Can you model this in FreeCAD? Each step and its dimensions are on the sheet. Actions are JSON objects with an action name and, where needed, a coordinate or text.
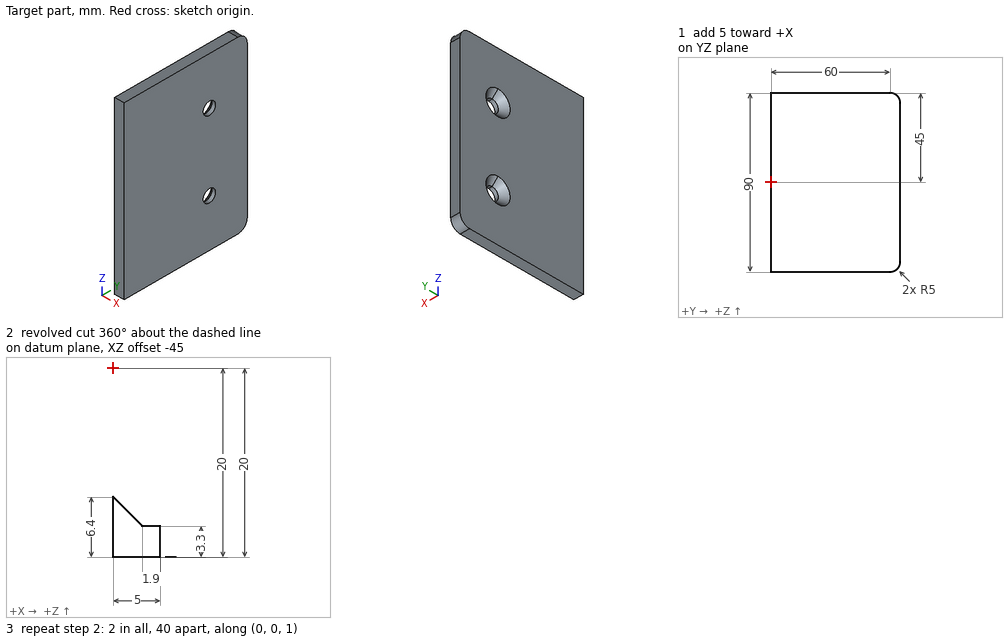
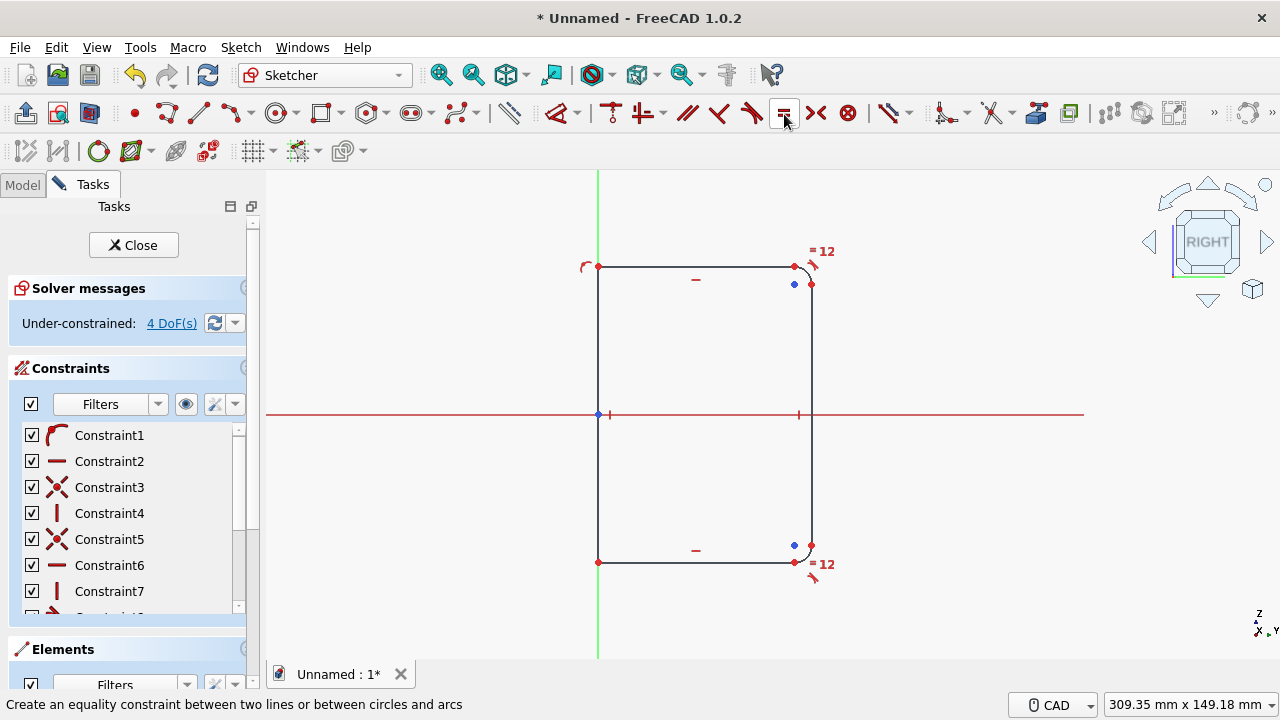
{"action": "left_click", "coordinate": [556, 114]}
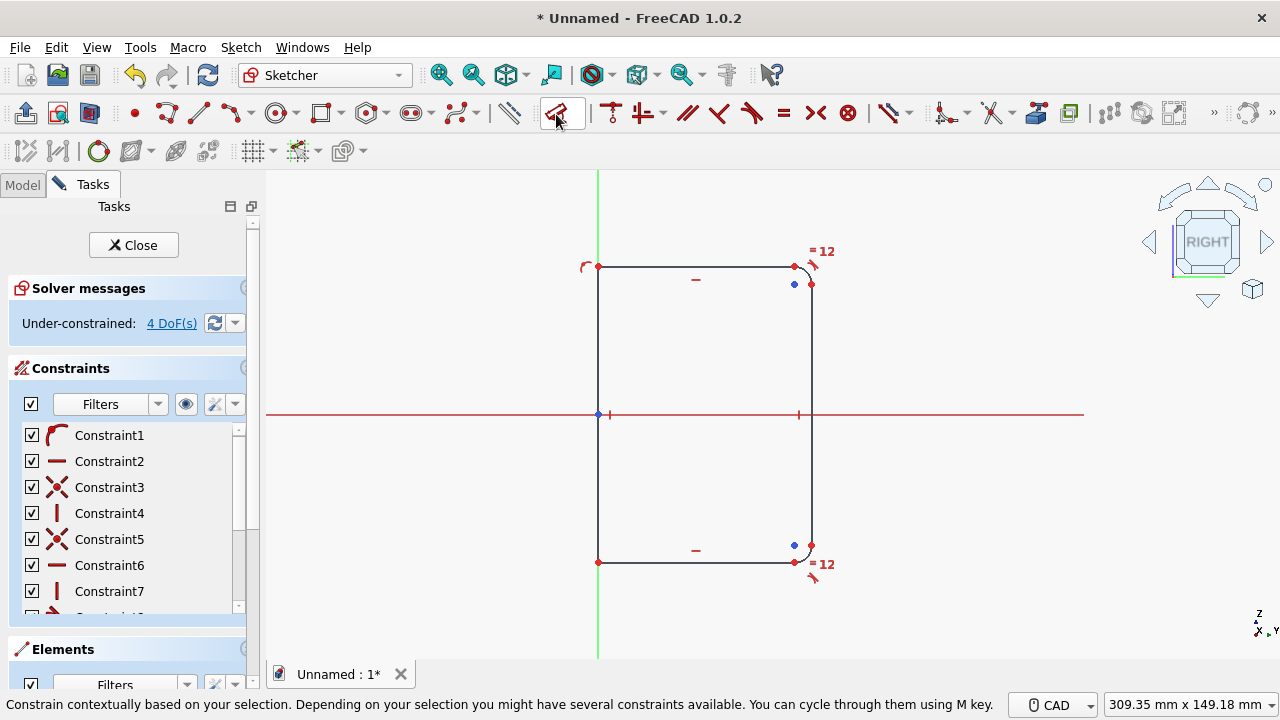
{"action": "scroll", "coordinate": [807, 558], "scroll_direction": "up", "scroll_amount": 5}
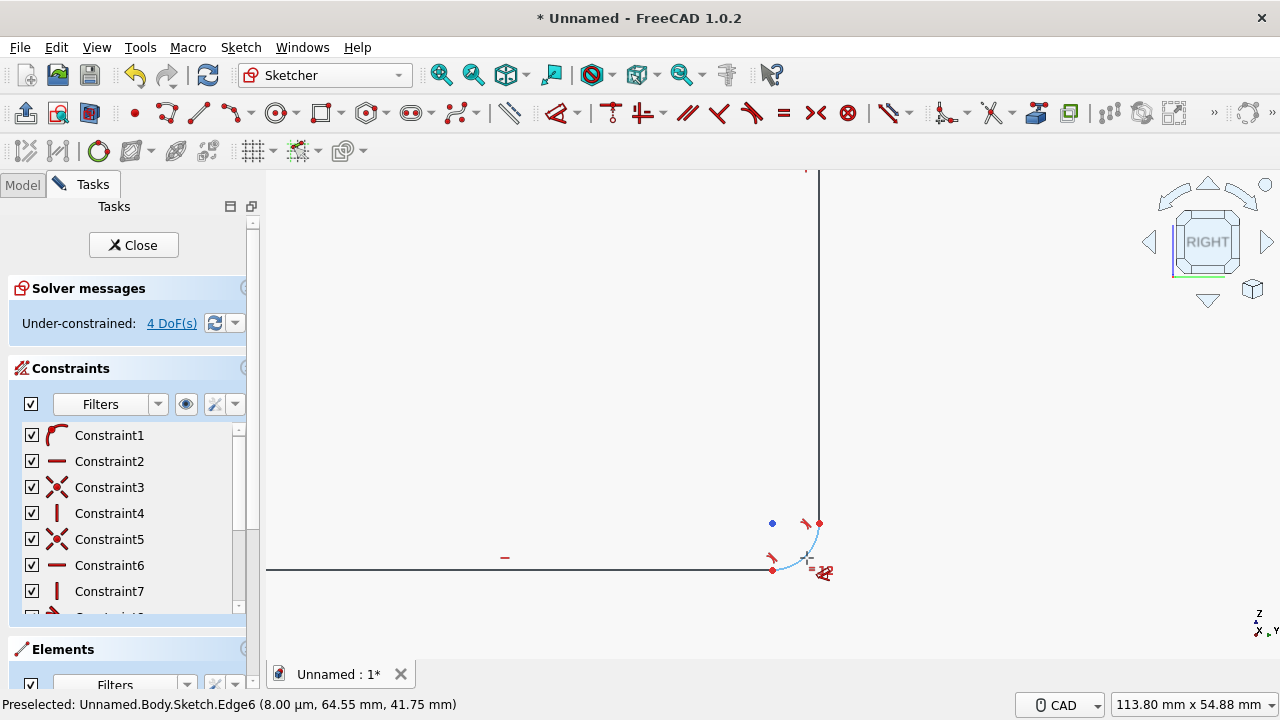
{"action": "left_click", "coordinate": [805, 556]}
{"action": "left_click", "coordinate": [828, 579]}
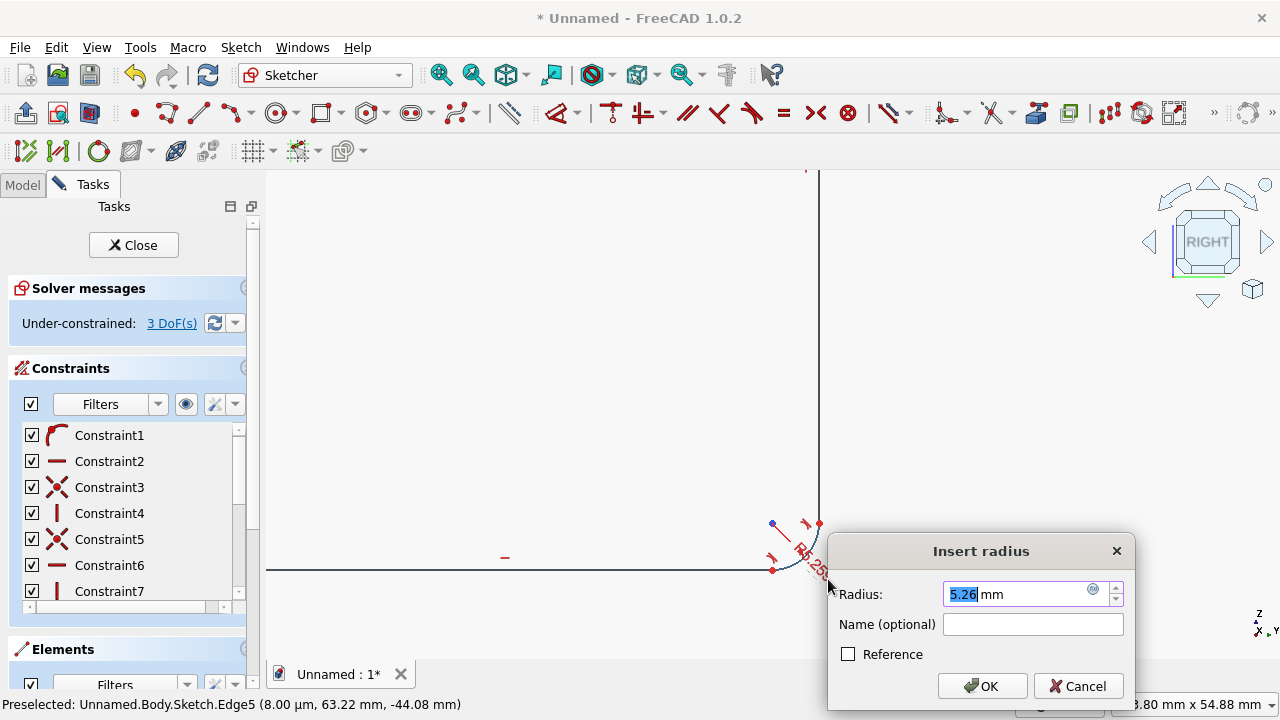
{"action": "type", "text": "5"}
{"action": "key", "text": "Return"}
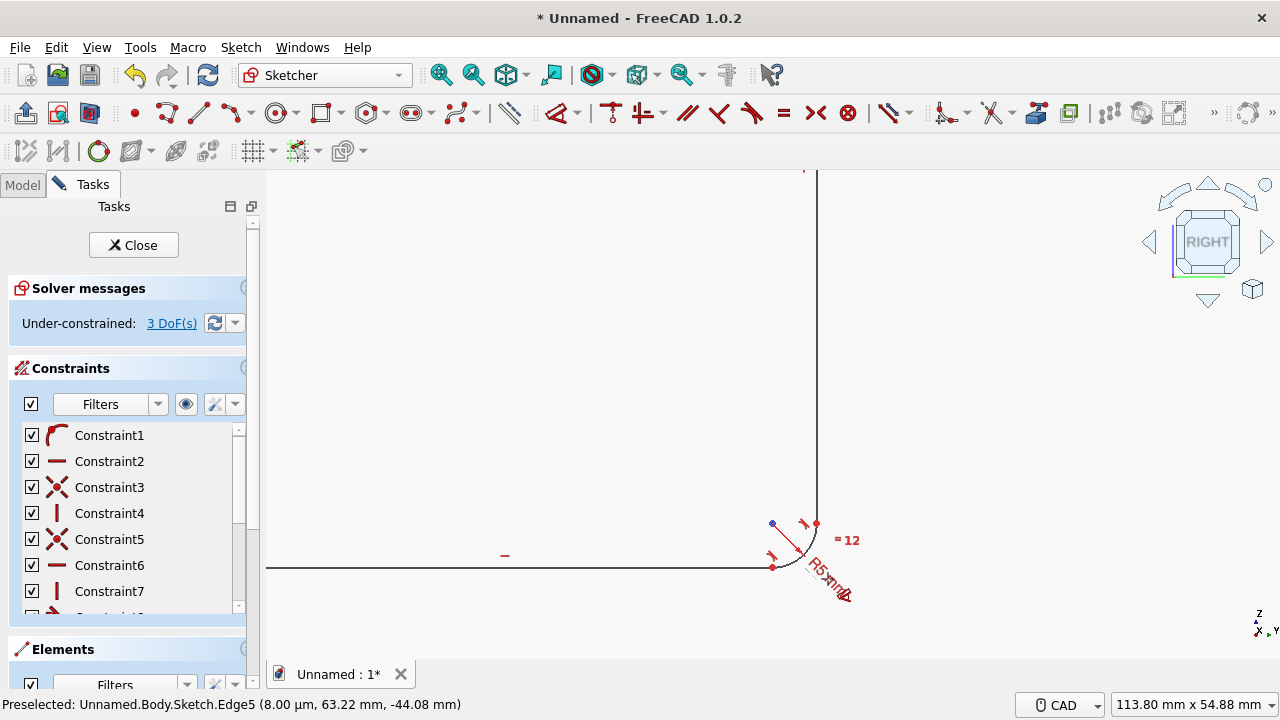
{"action": "scroll", "coordinate": [807, 559], "scroll_direction": "down", "scroll_amount": 5}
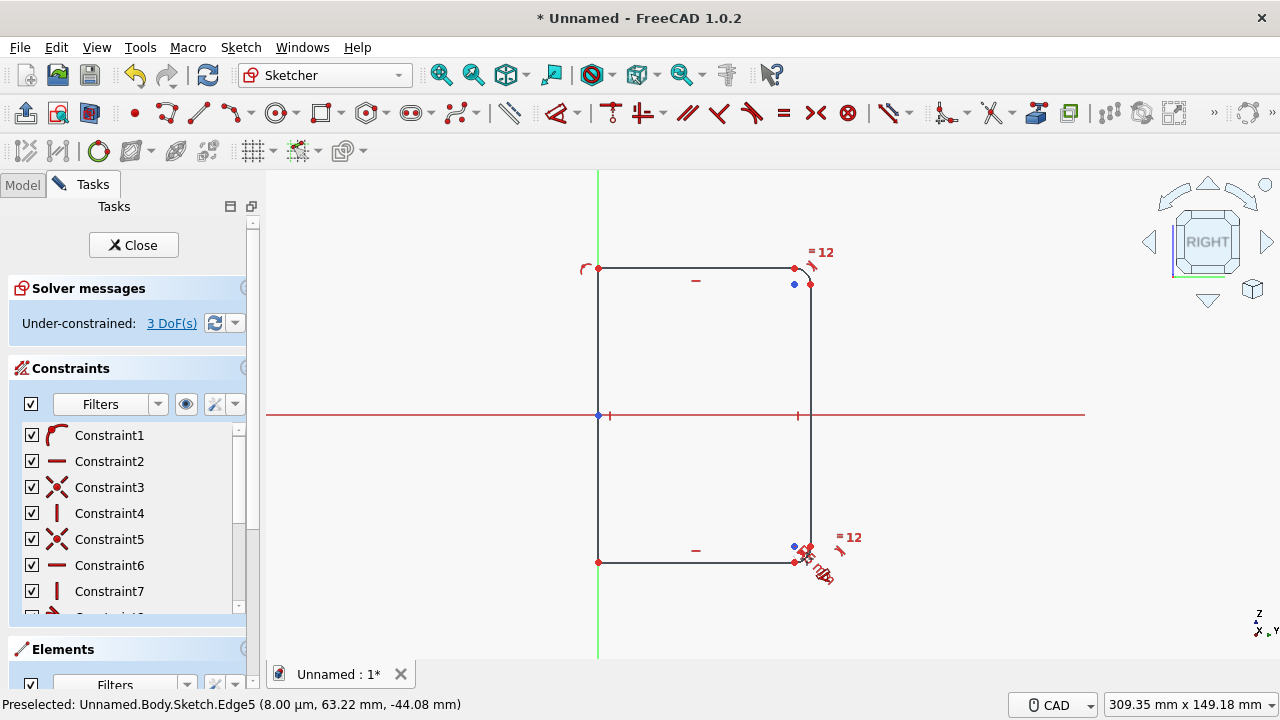
{"action": "left_click", "coordinate": [736, 268]}
{"action": "left_click", "coordinate": [696, 234]}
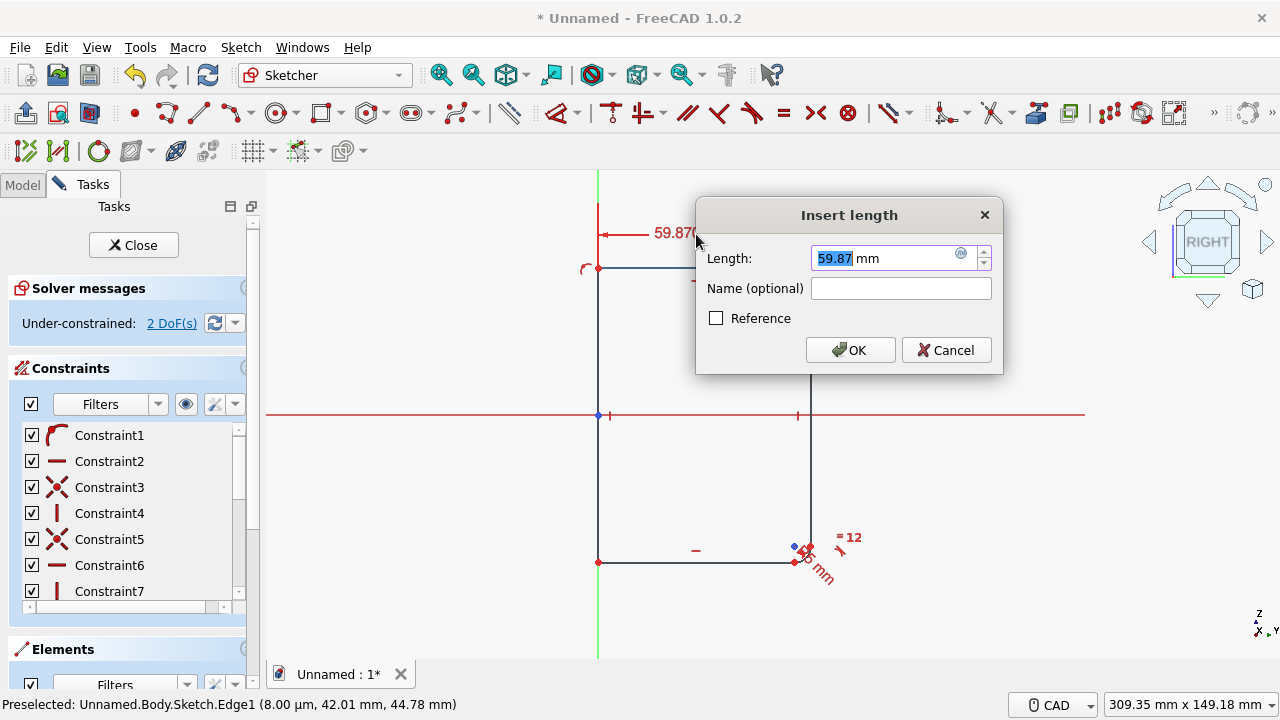
{"action": "type", "text": "60"}
{"action": "key", "text": "Return"}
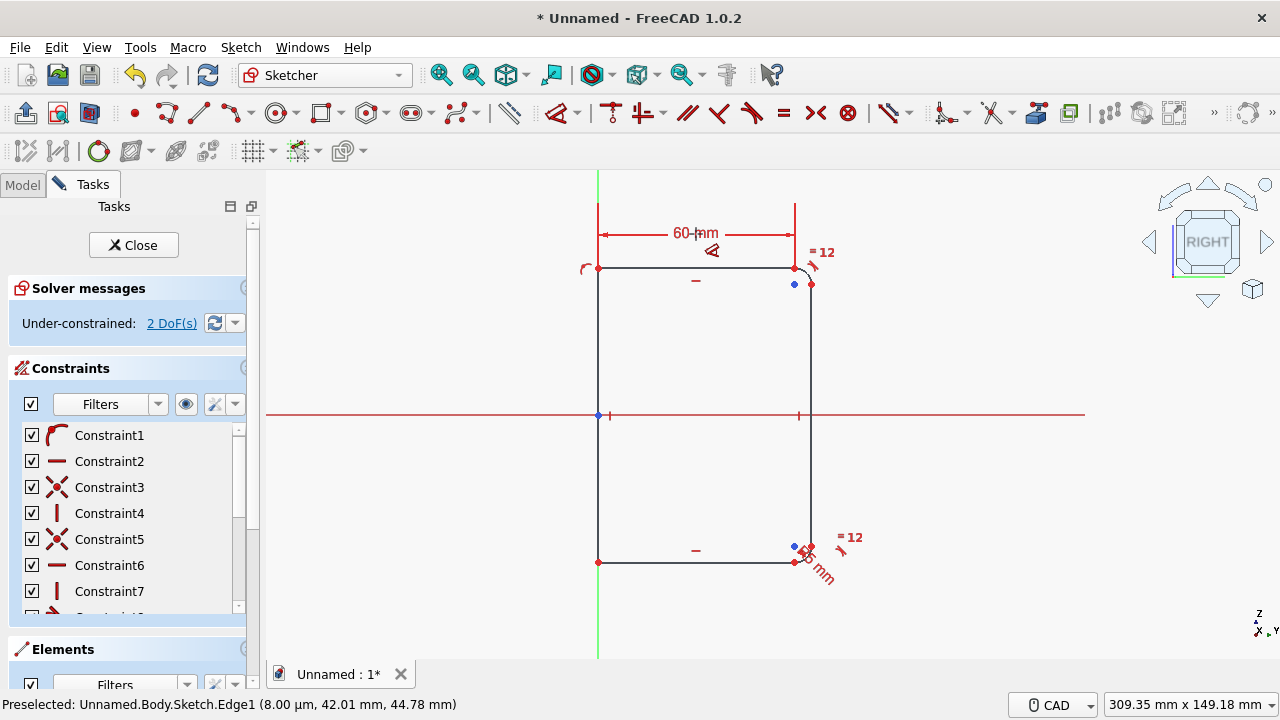
{"action": "left_click", "coordinate": [598, 357]}
{"action": "left_click", "coordinate": [564, 348]}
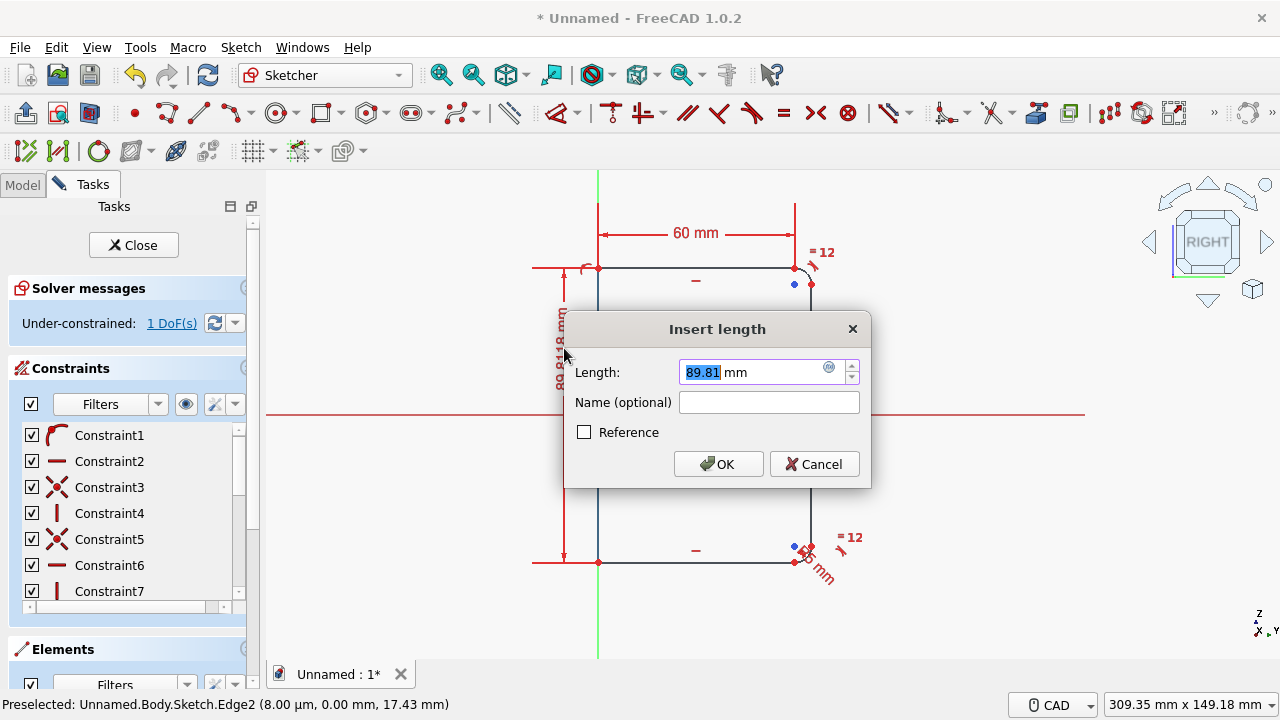
{"action": "type", "text": "90"}
{"action": "key", "text": "Return"}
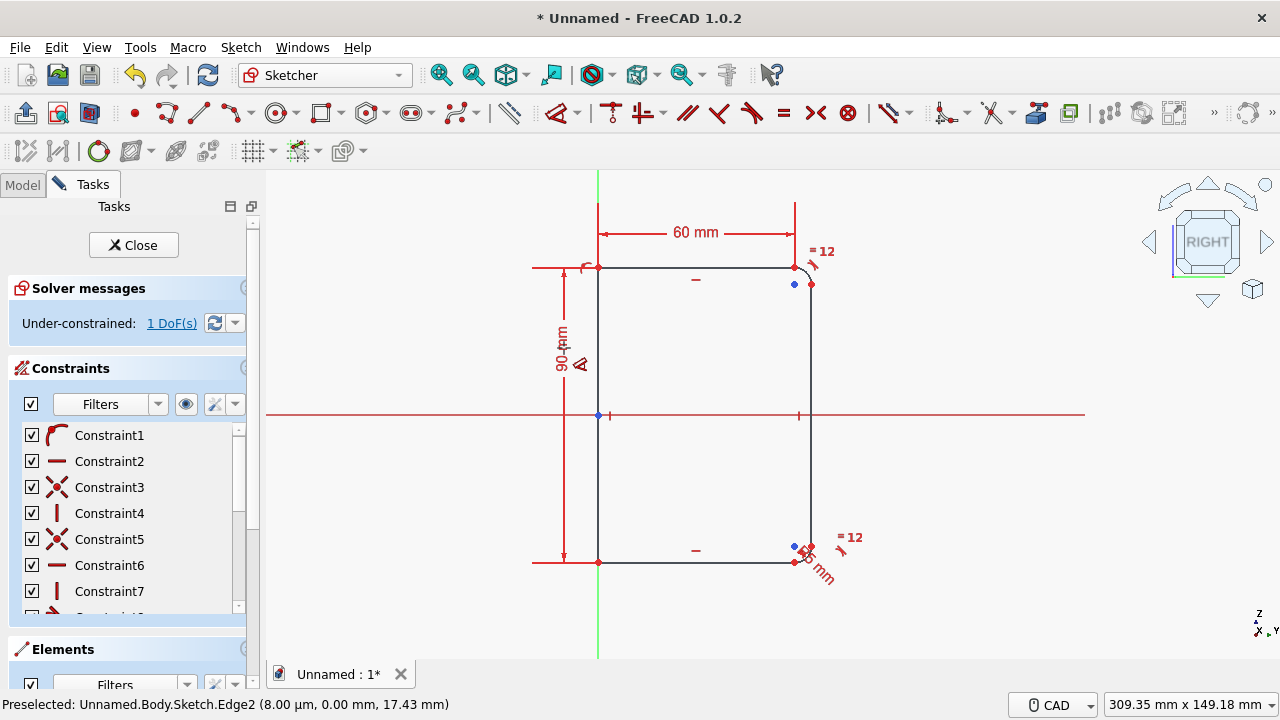
{"action": "left_click", "coordinate": [795, 268]}
{"action": "left_click", "coordinate": [564, 308]}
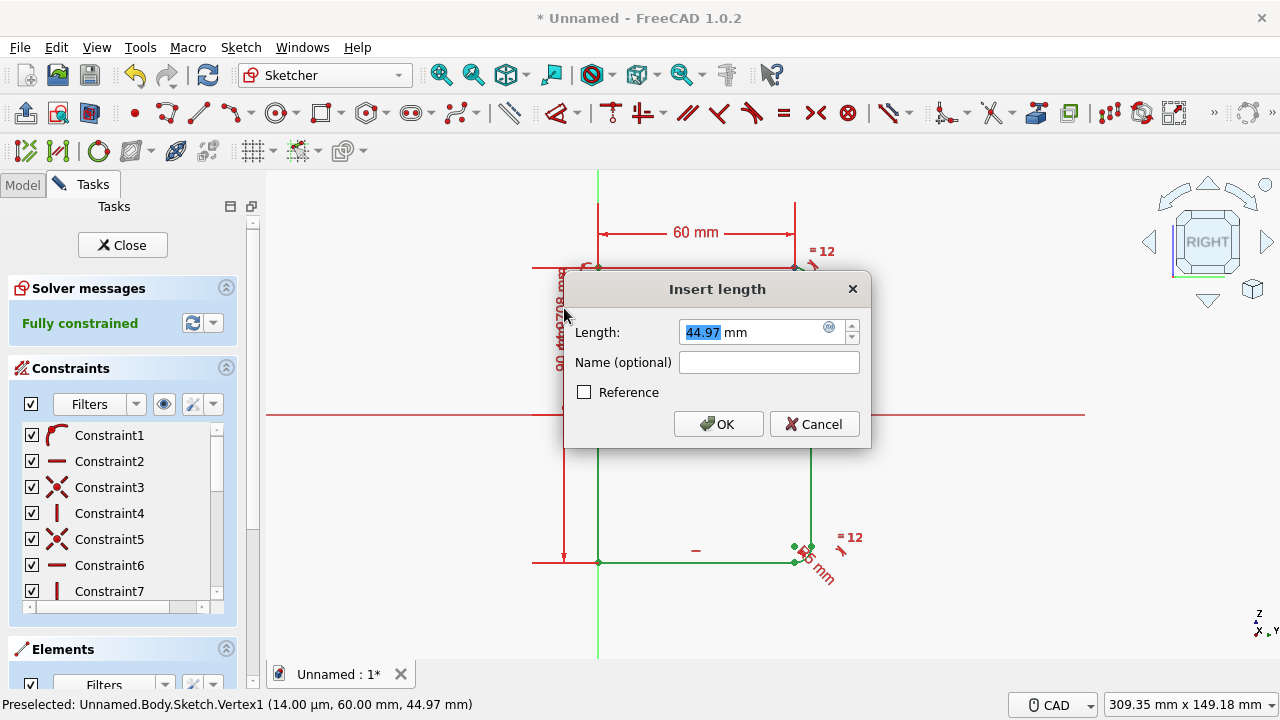
{"action": "type", "text": "45"}
{"action": "key", "text": "Return"}
{"action": "key", "text": "Escape"}